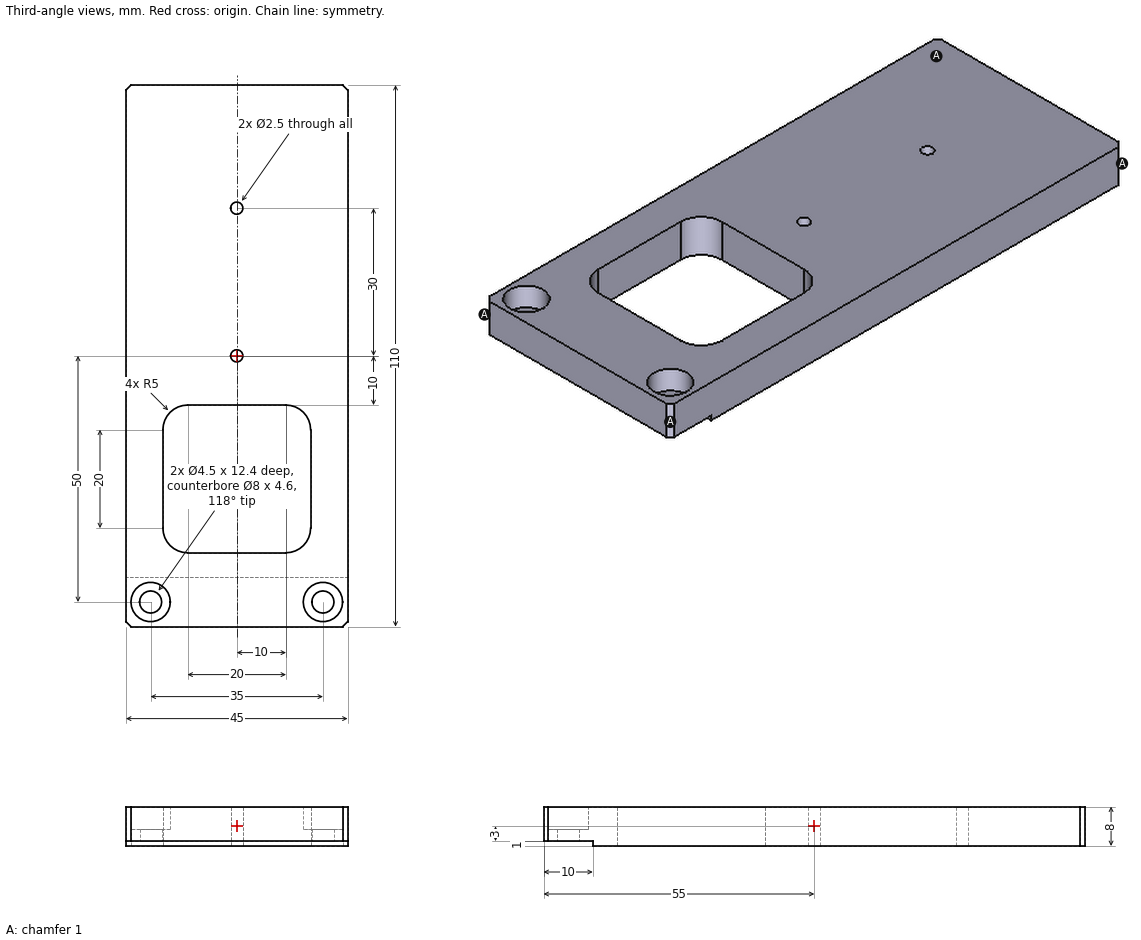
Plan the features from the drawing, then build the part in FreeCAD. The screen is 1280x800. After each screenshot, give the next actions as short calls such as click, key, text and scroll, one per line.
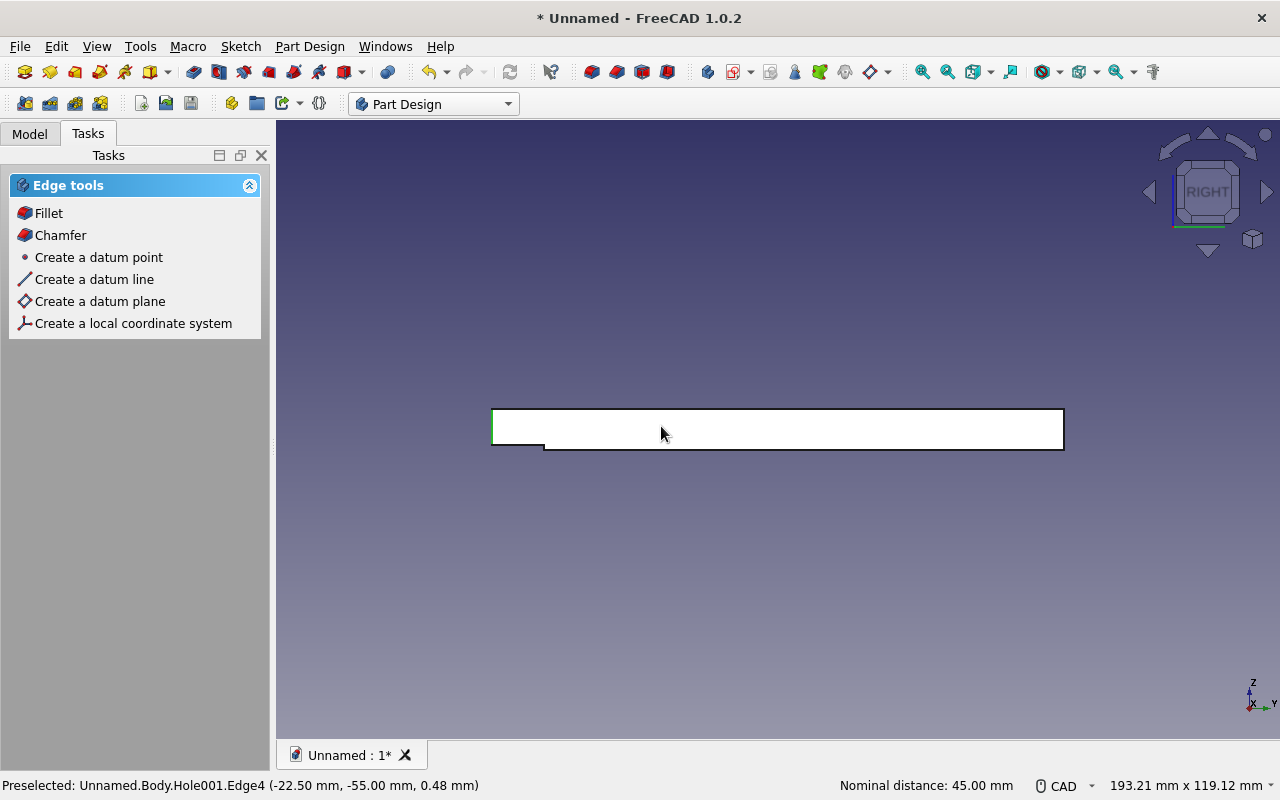
click(1064, 428, ctrl)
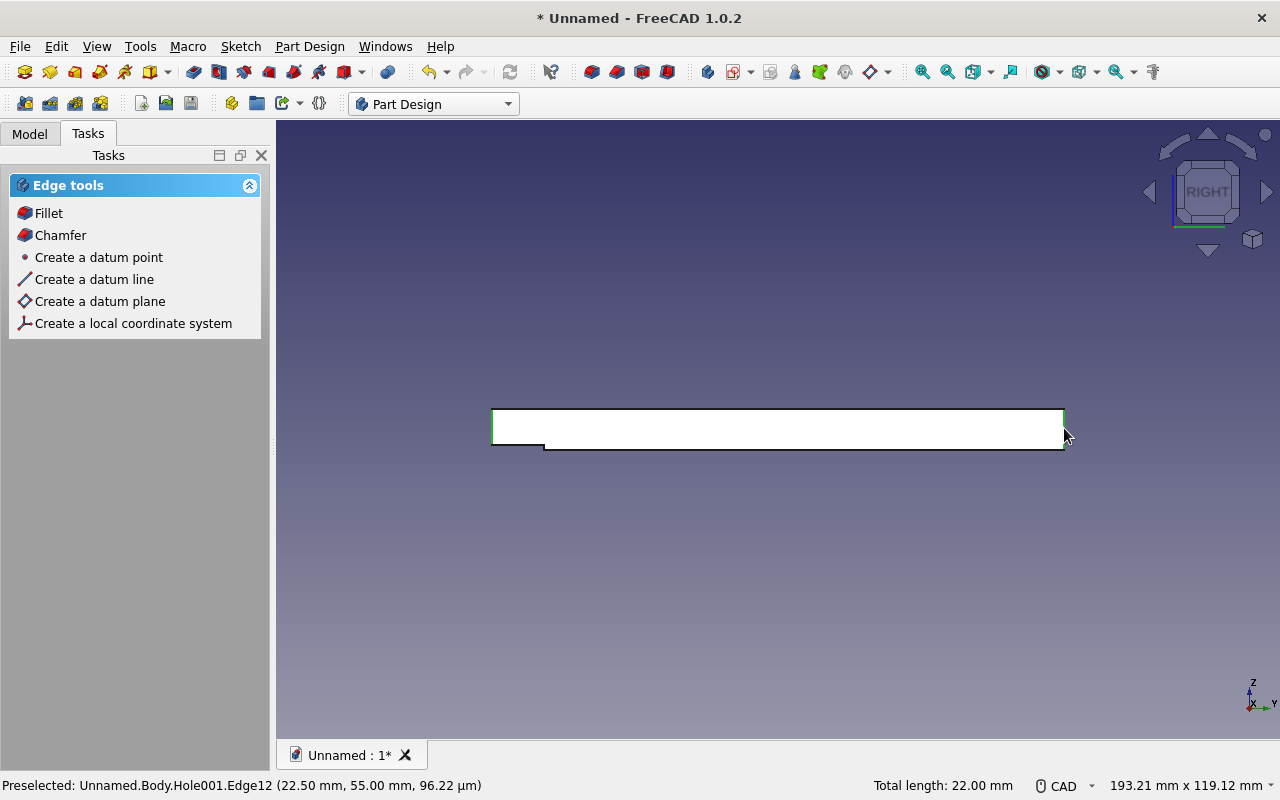
key(5)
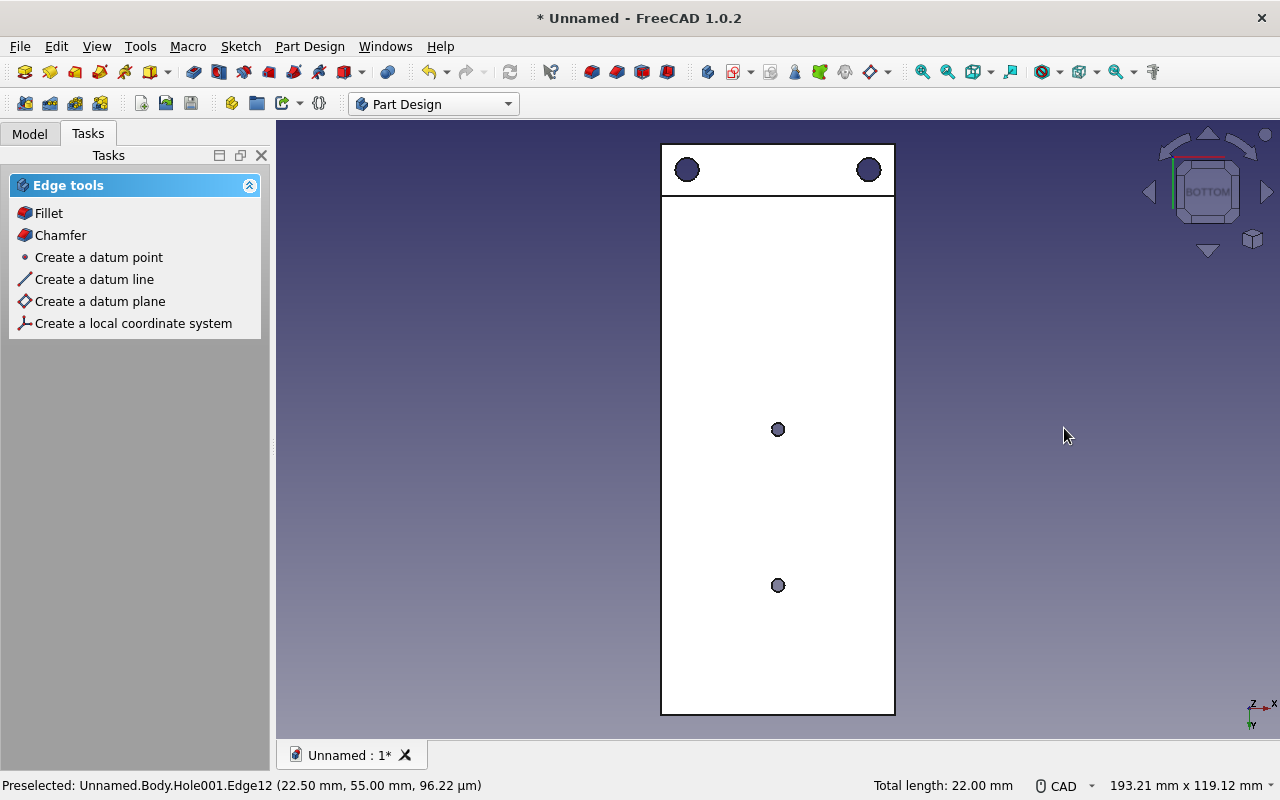
key(4)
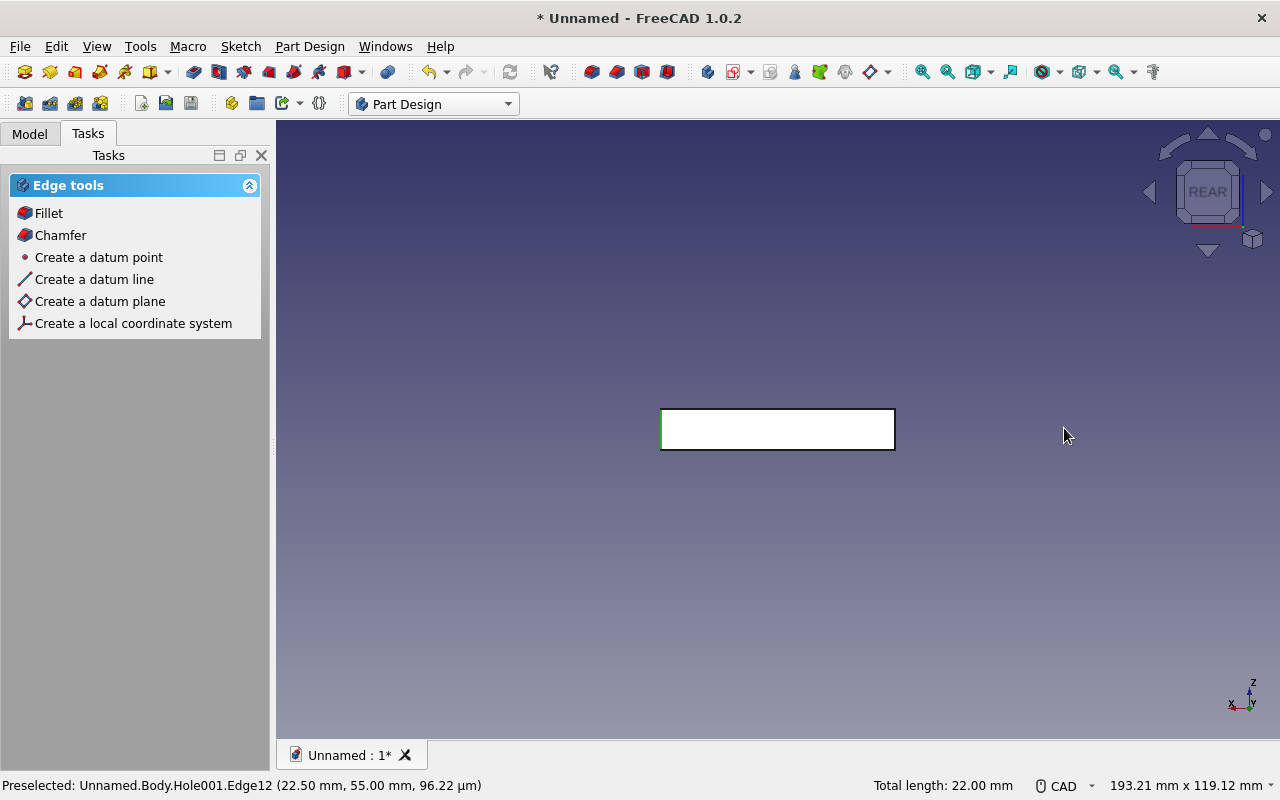
click(923, 72)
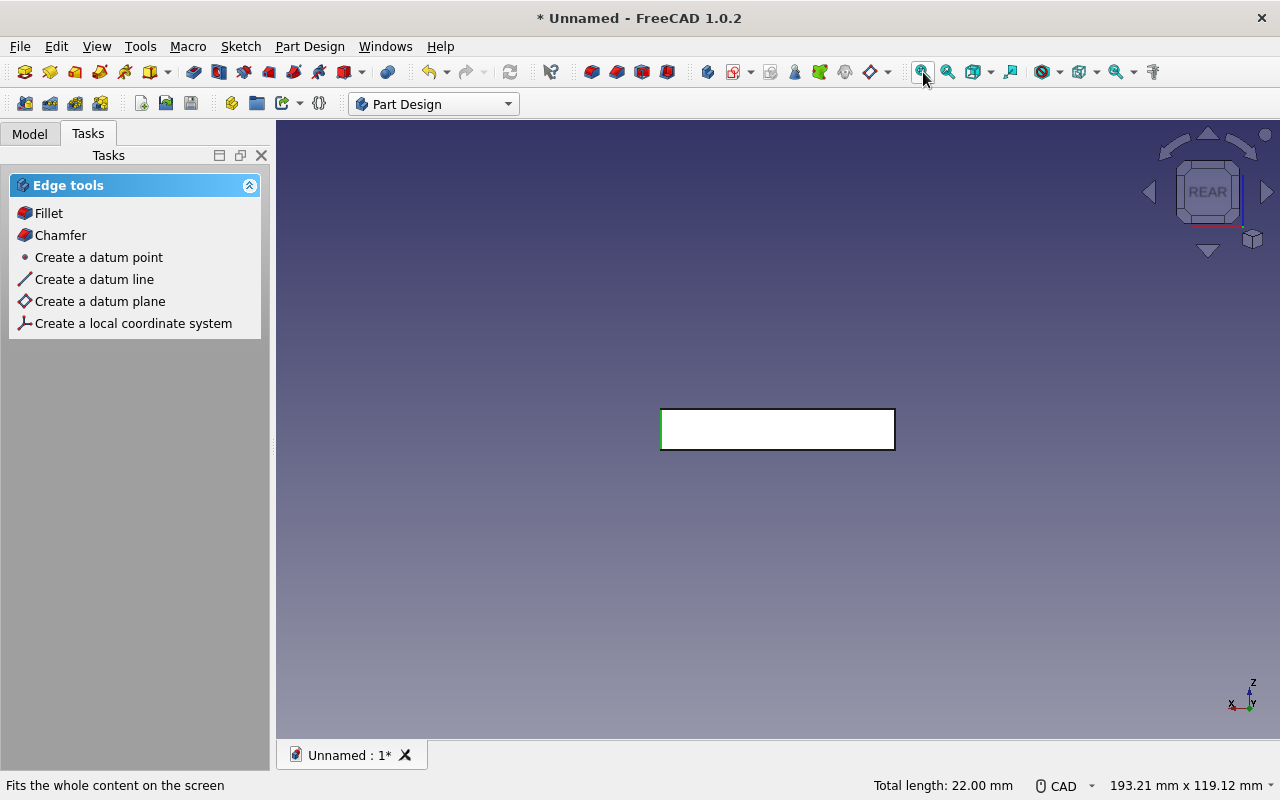
click(895, 429, ctrl)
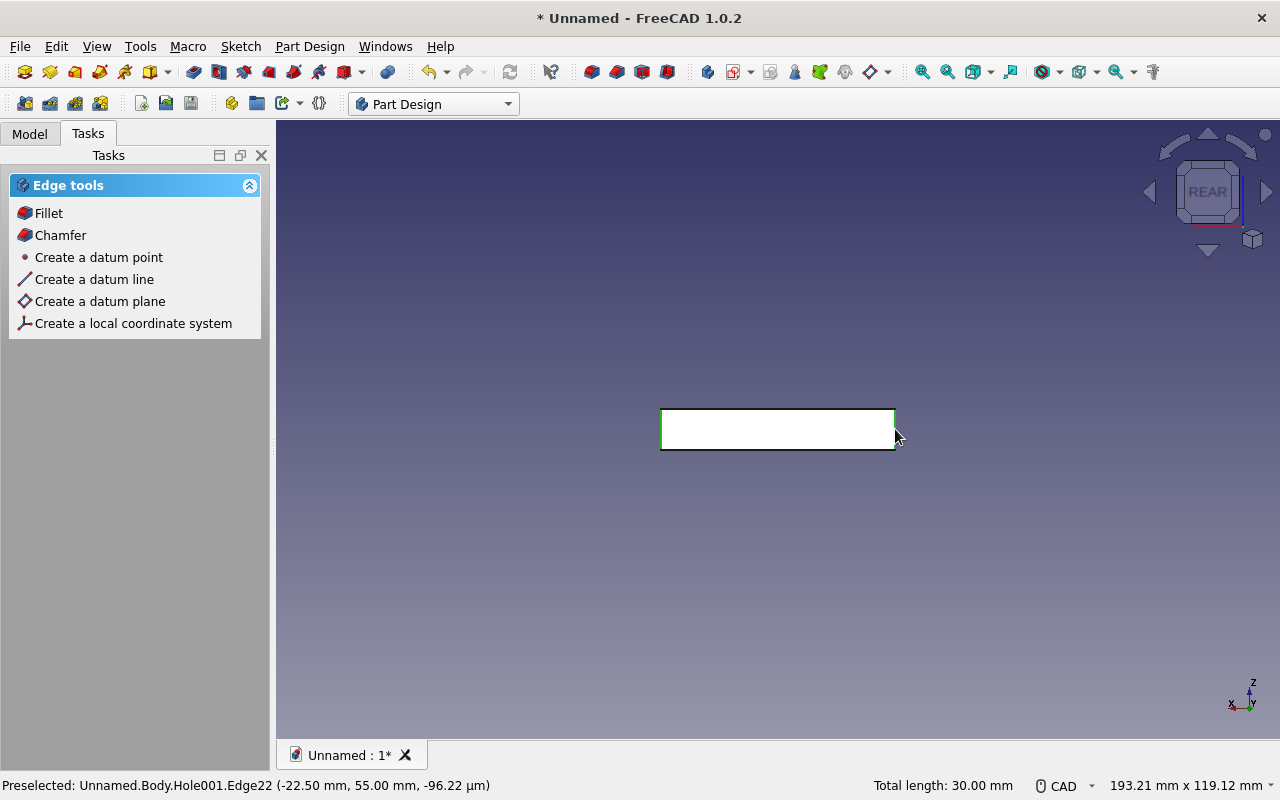
click(617, 72)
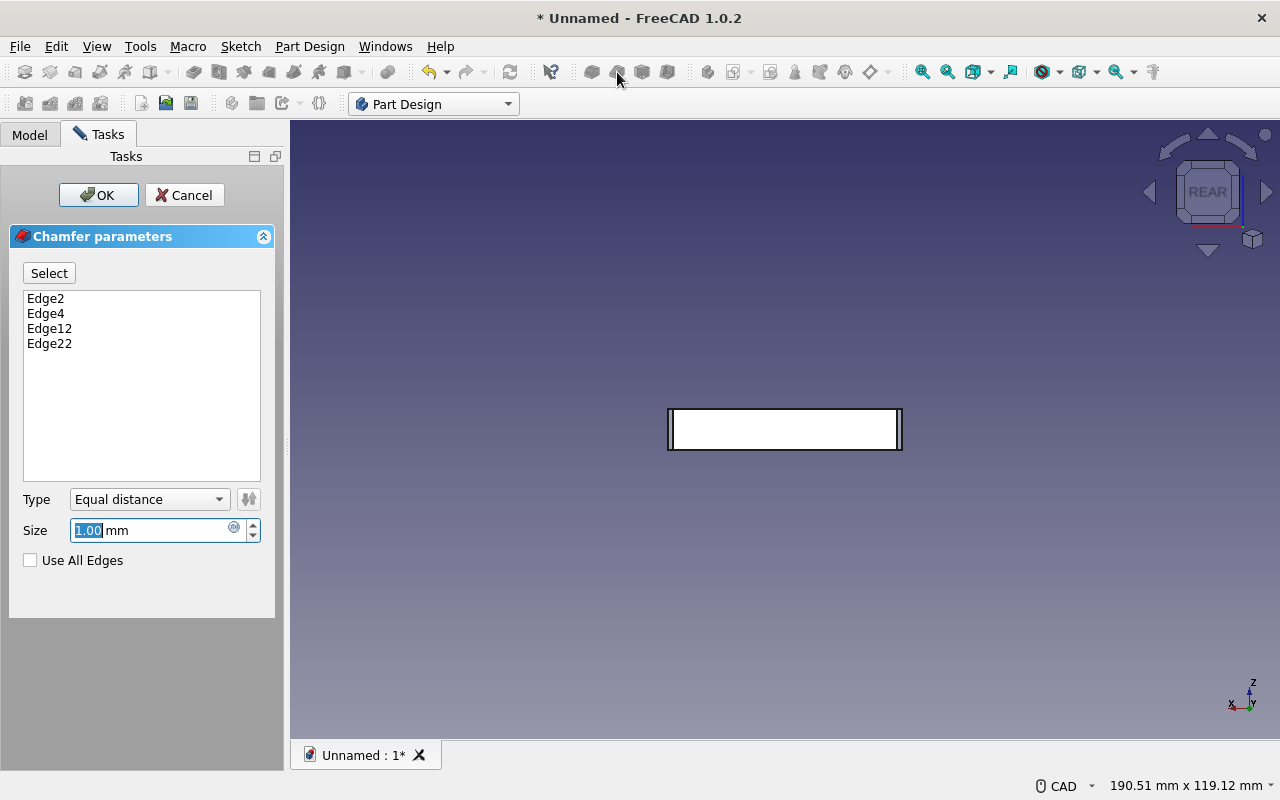
text(1)
key(Tab)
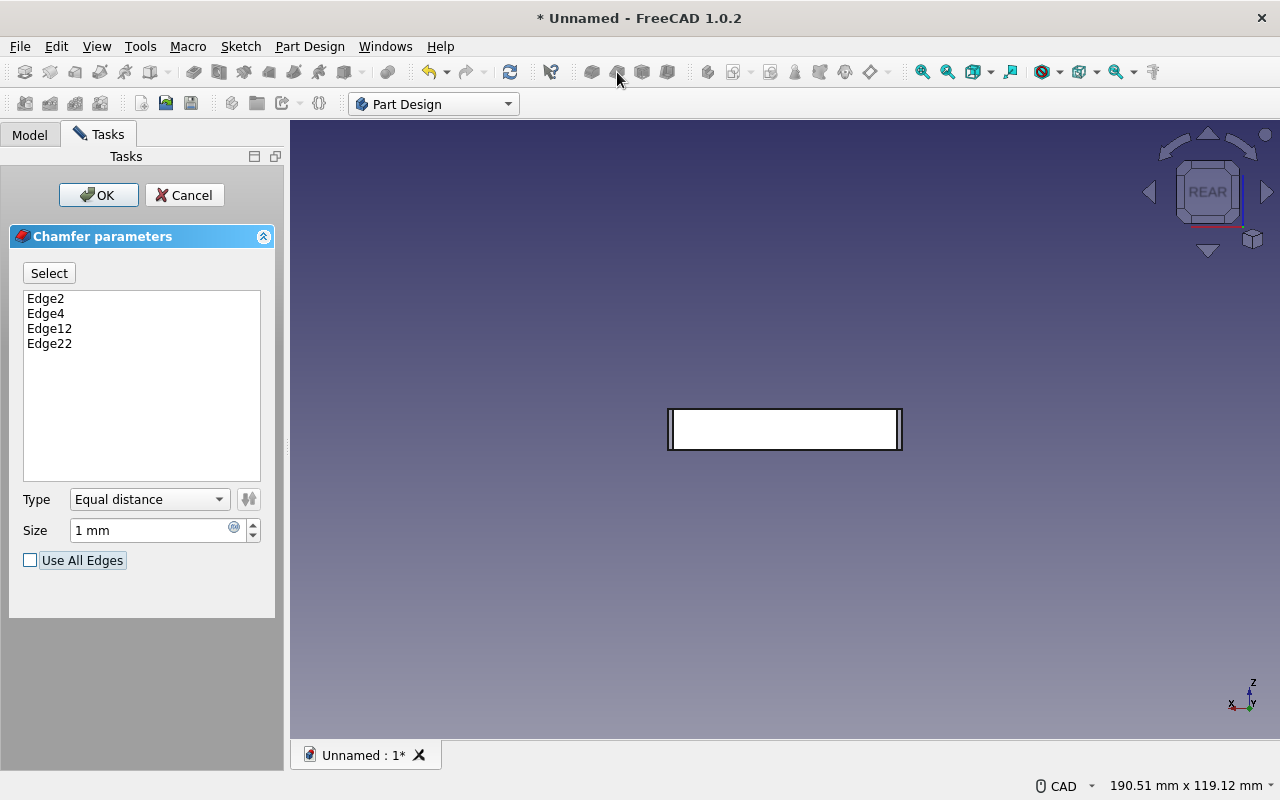
click(99, 195)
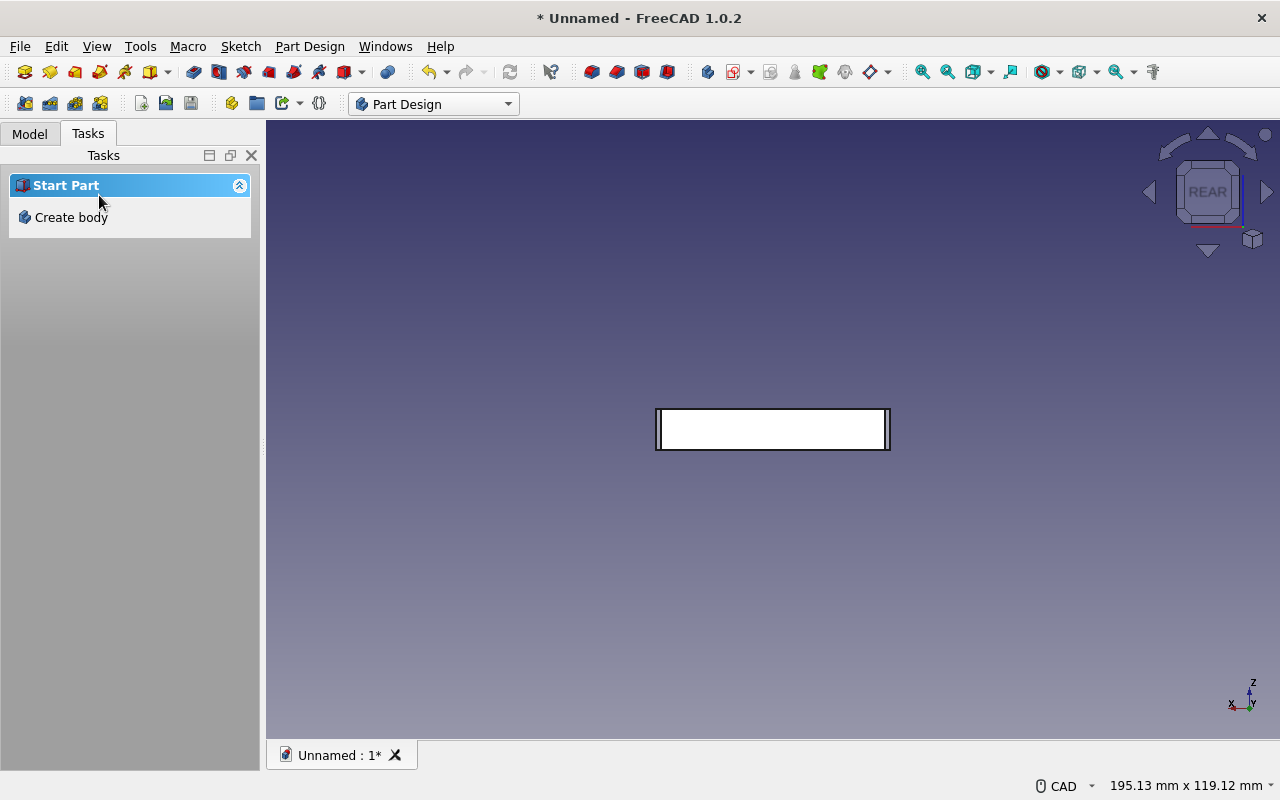
click(923, 72)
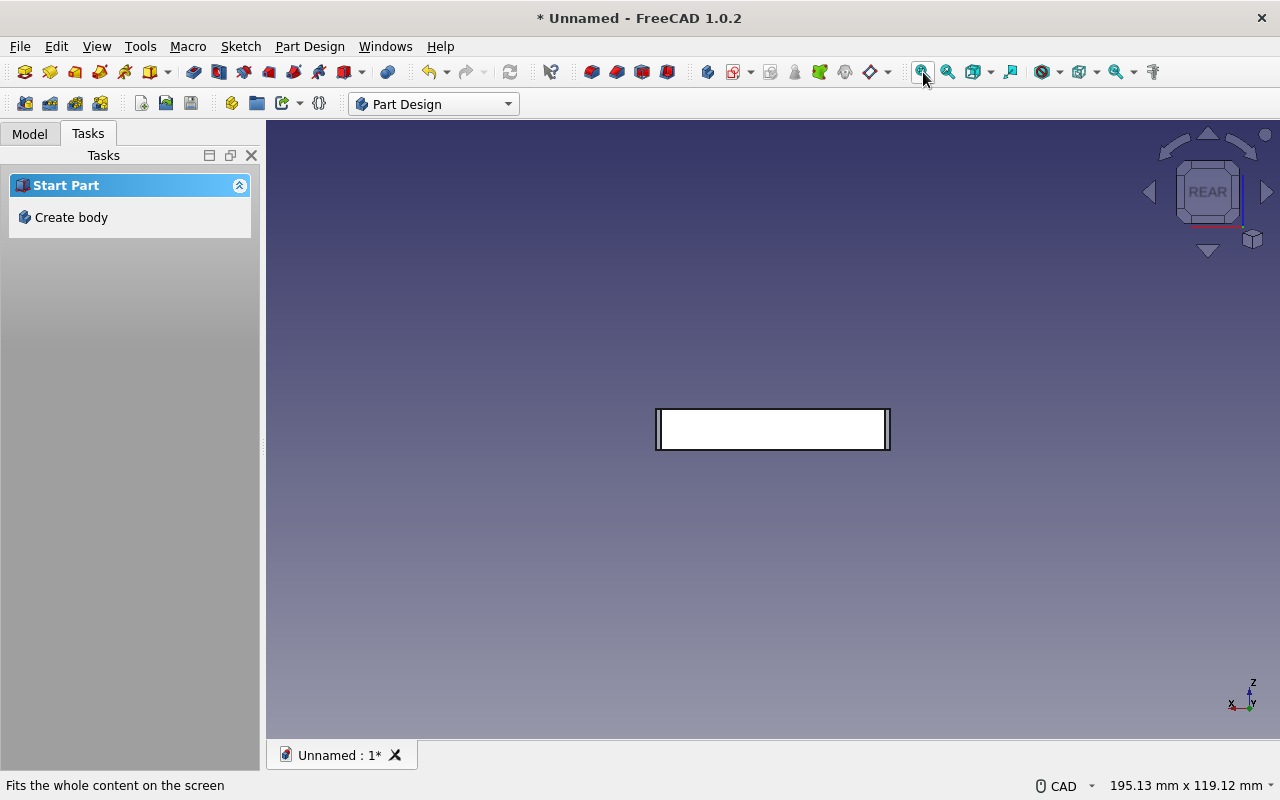
key(0)